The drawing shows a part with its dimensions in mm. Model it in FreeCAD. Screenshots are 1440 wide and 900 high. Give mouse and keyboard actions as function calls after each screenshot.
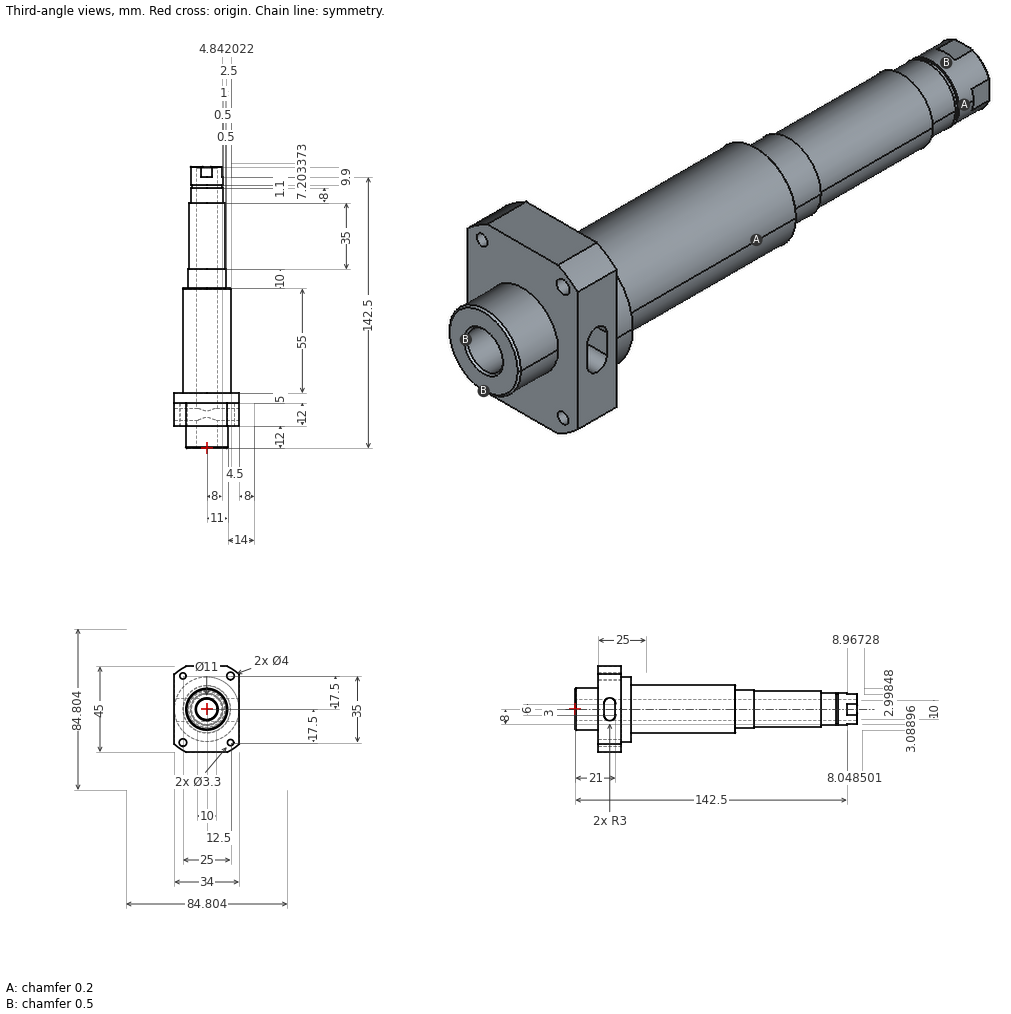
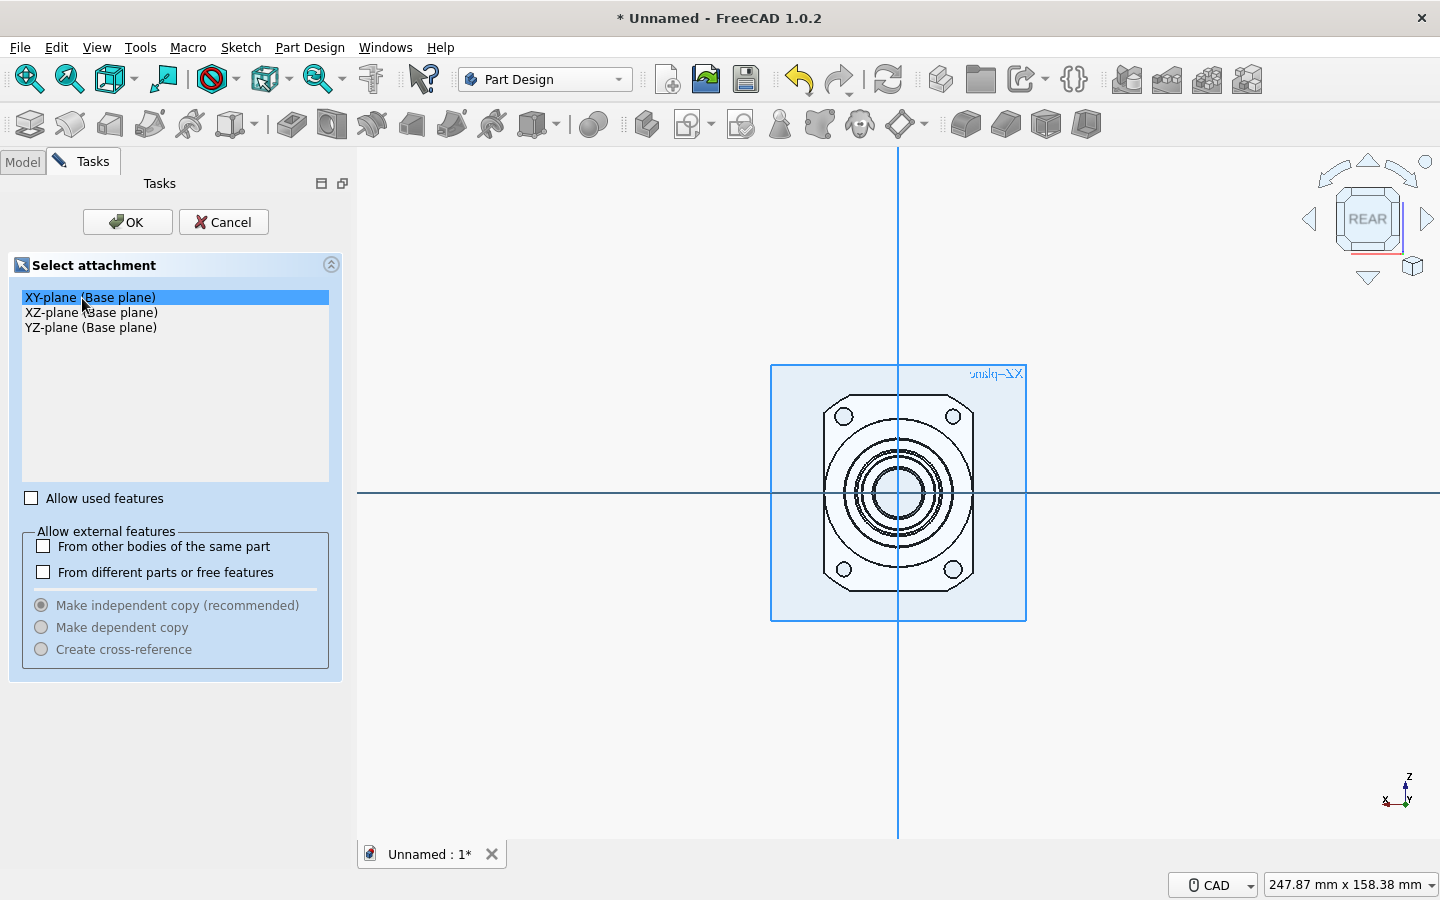
click(128, 222)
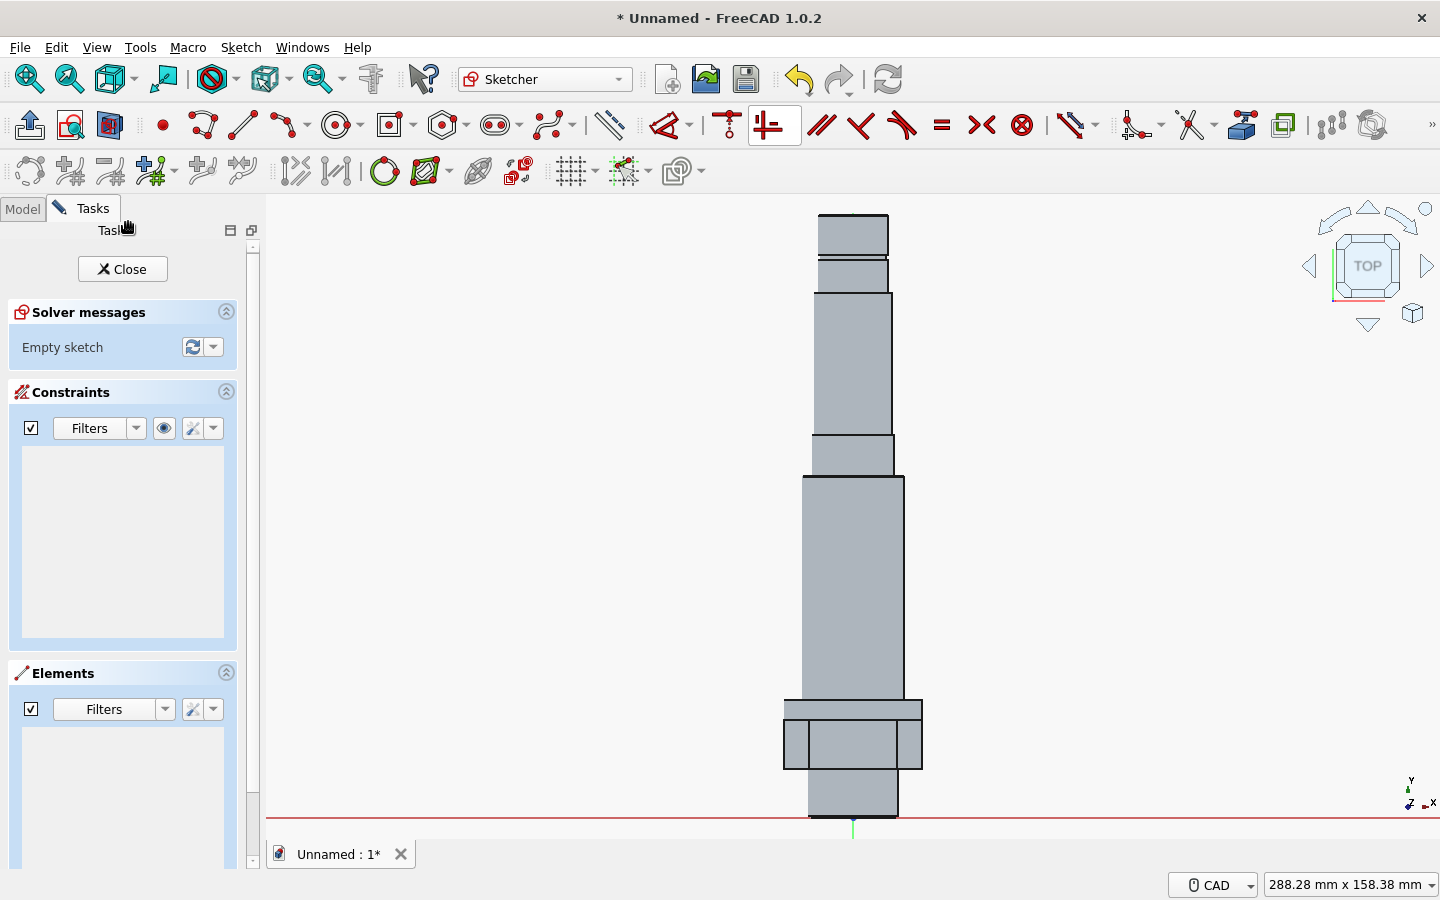
click(110, 126)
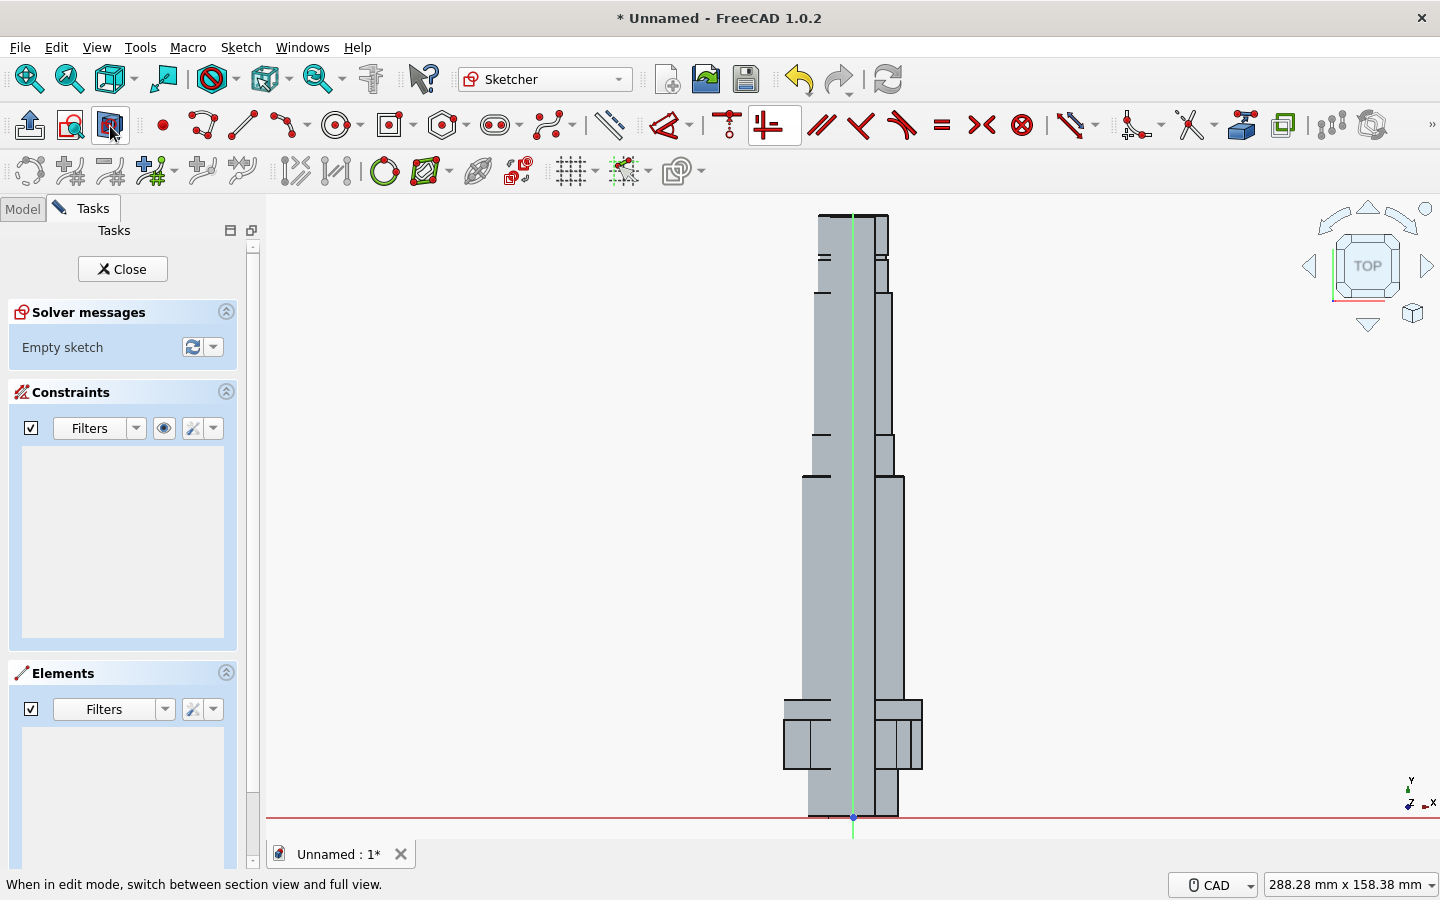
scroll(784, 516, down, 5)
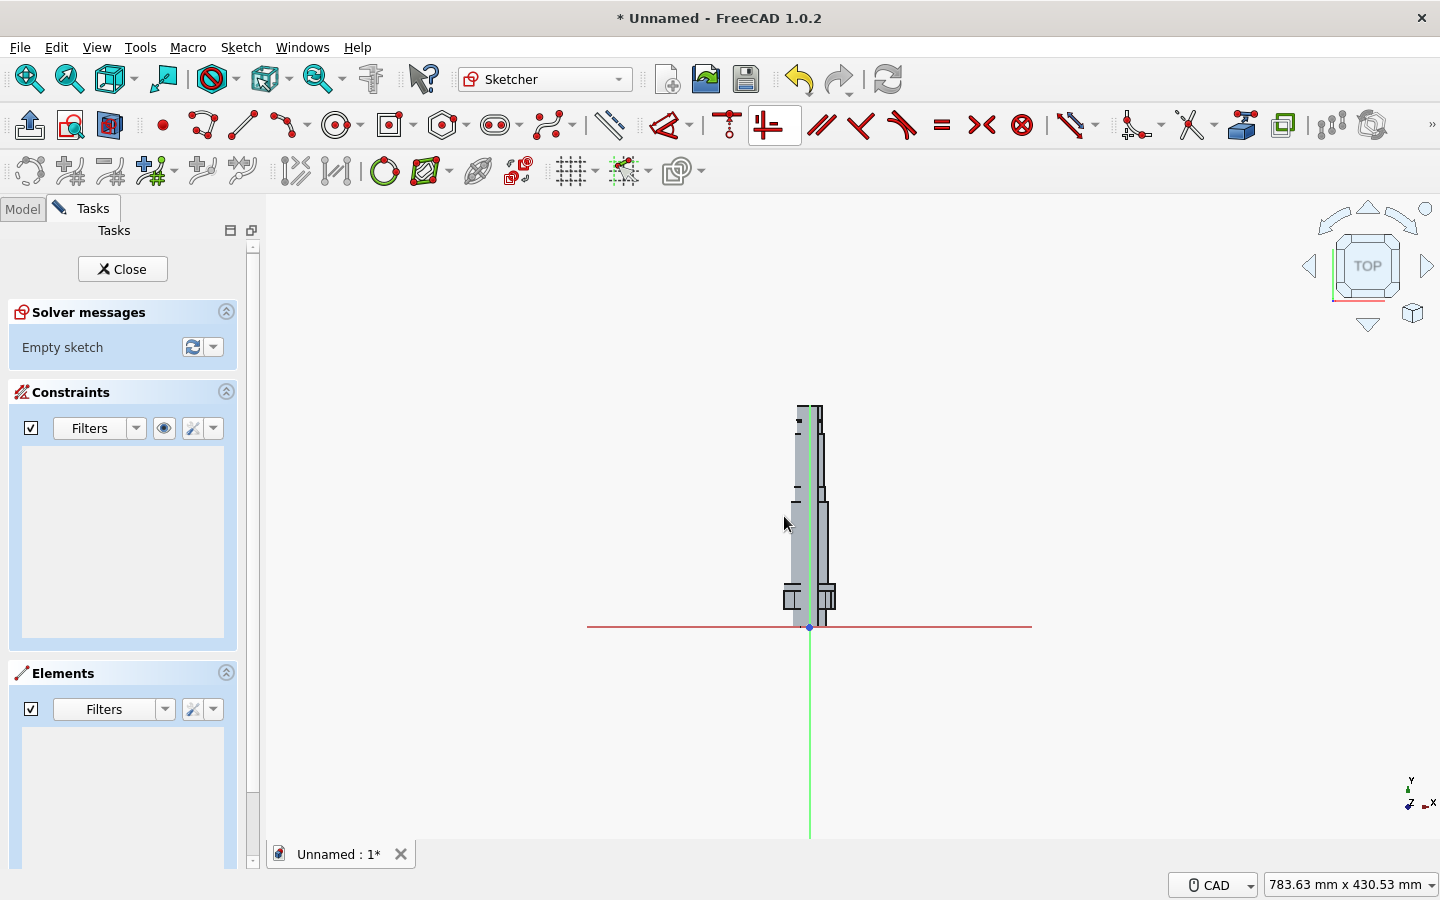
scroll(827, 403, up, 15)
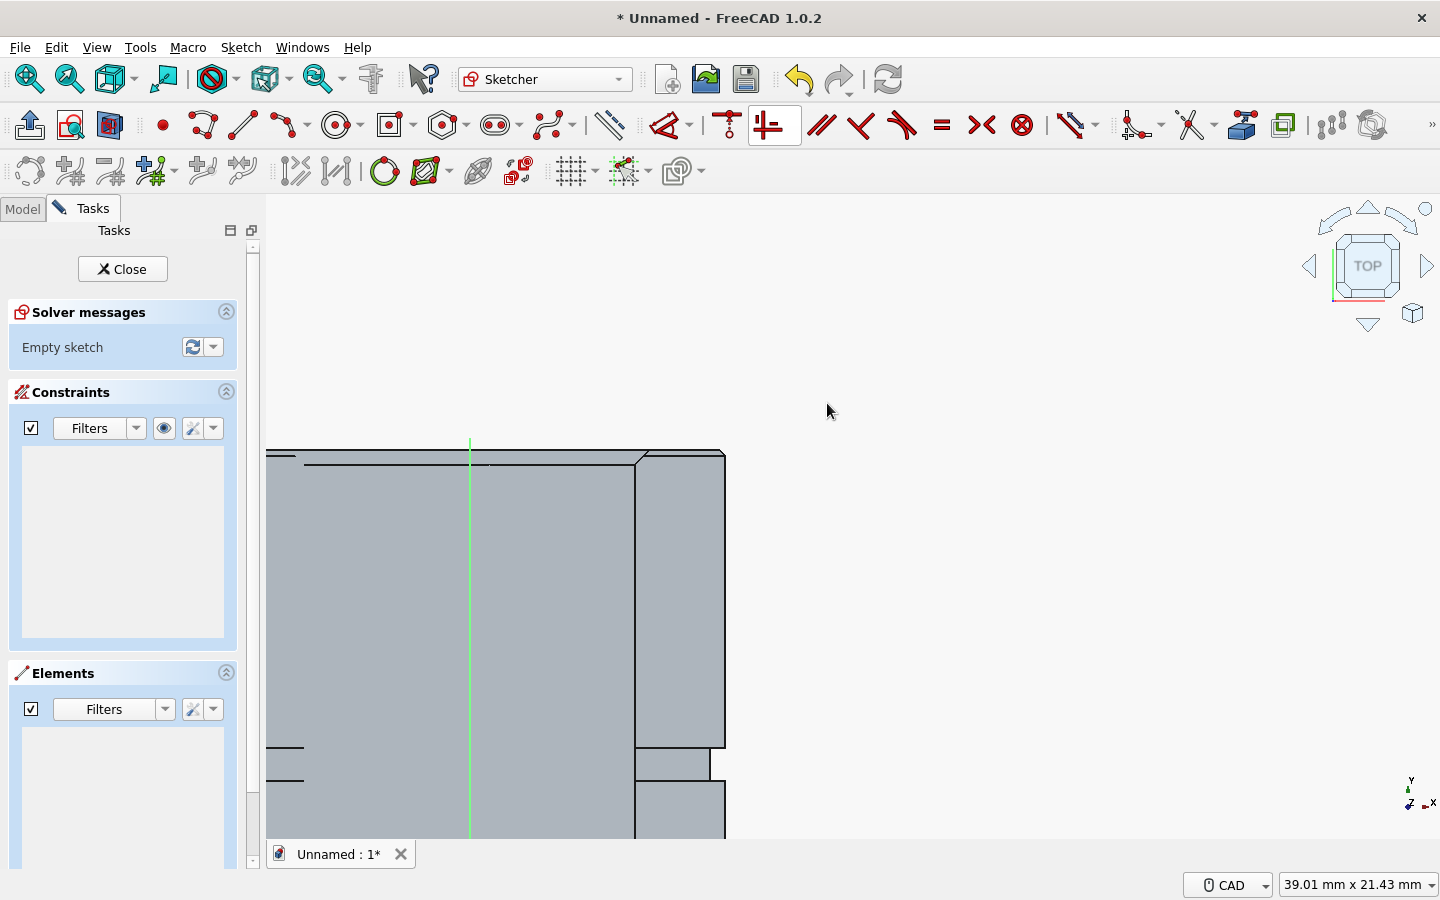
scroll(782, 495, up, 3)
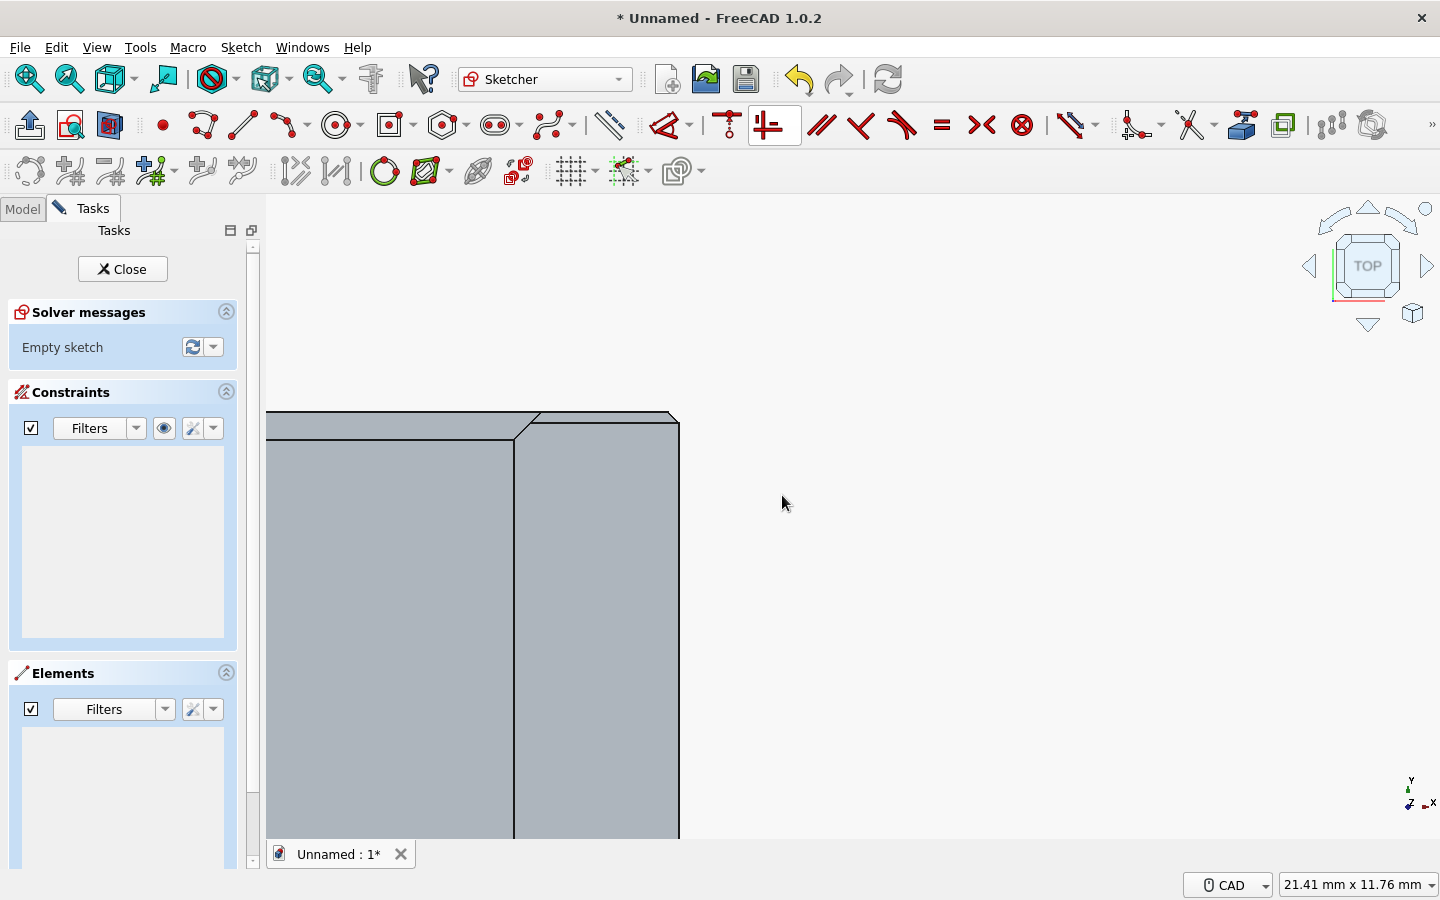
key(g)
key(r)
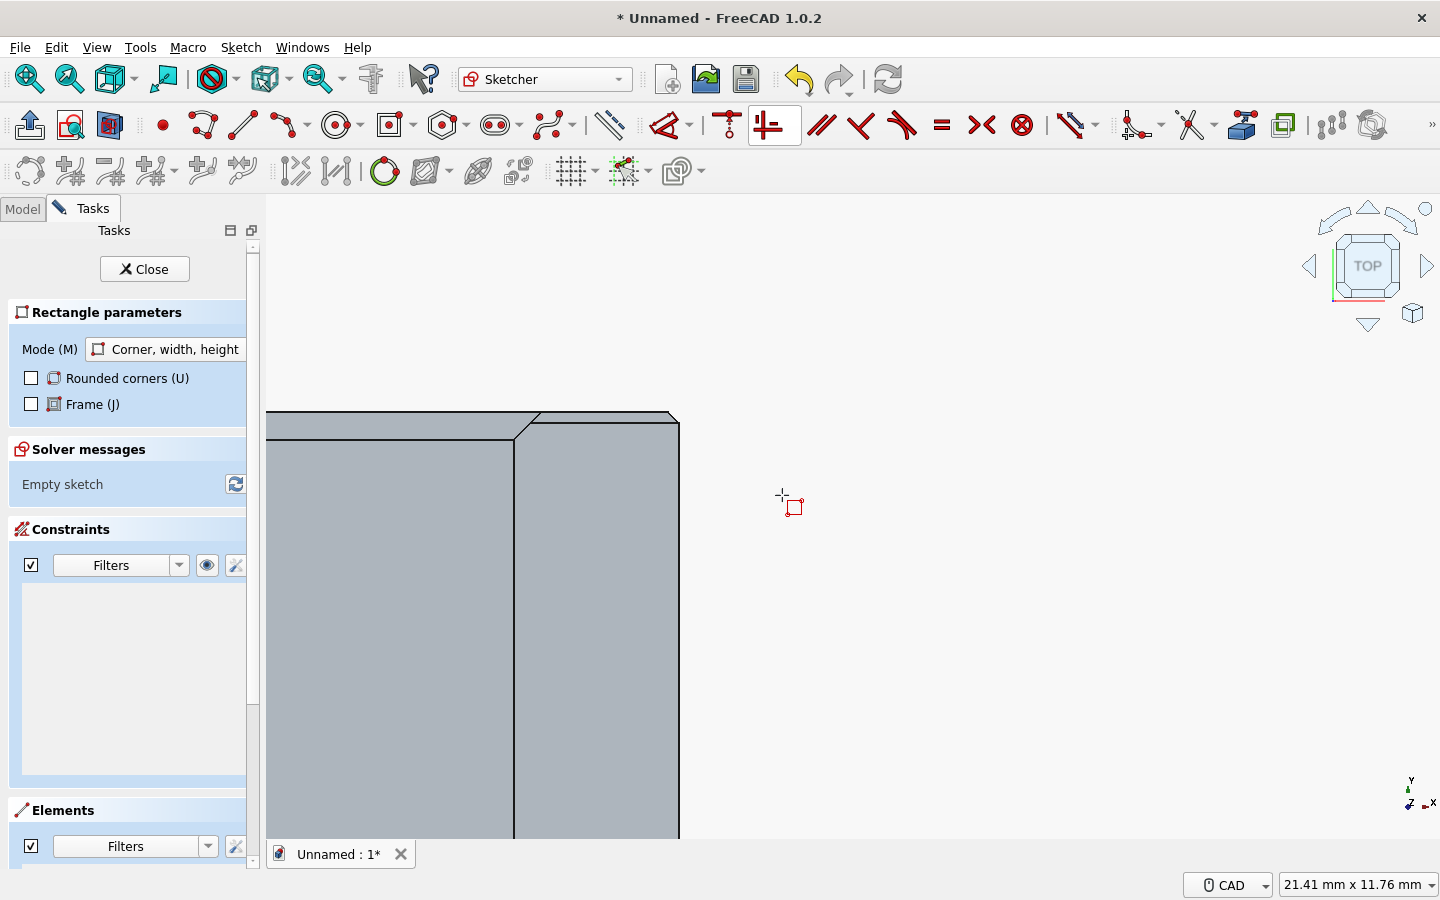
click(651, 319)
move(917, 714)